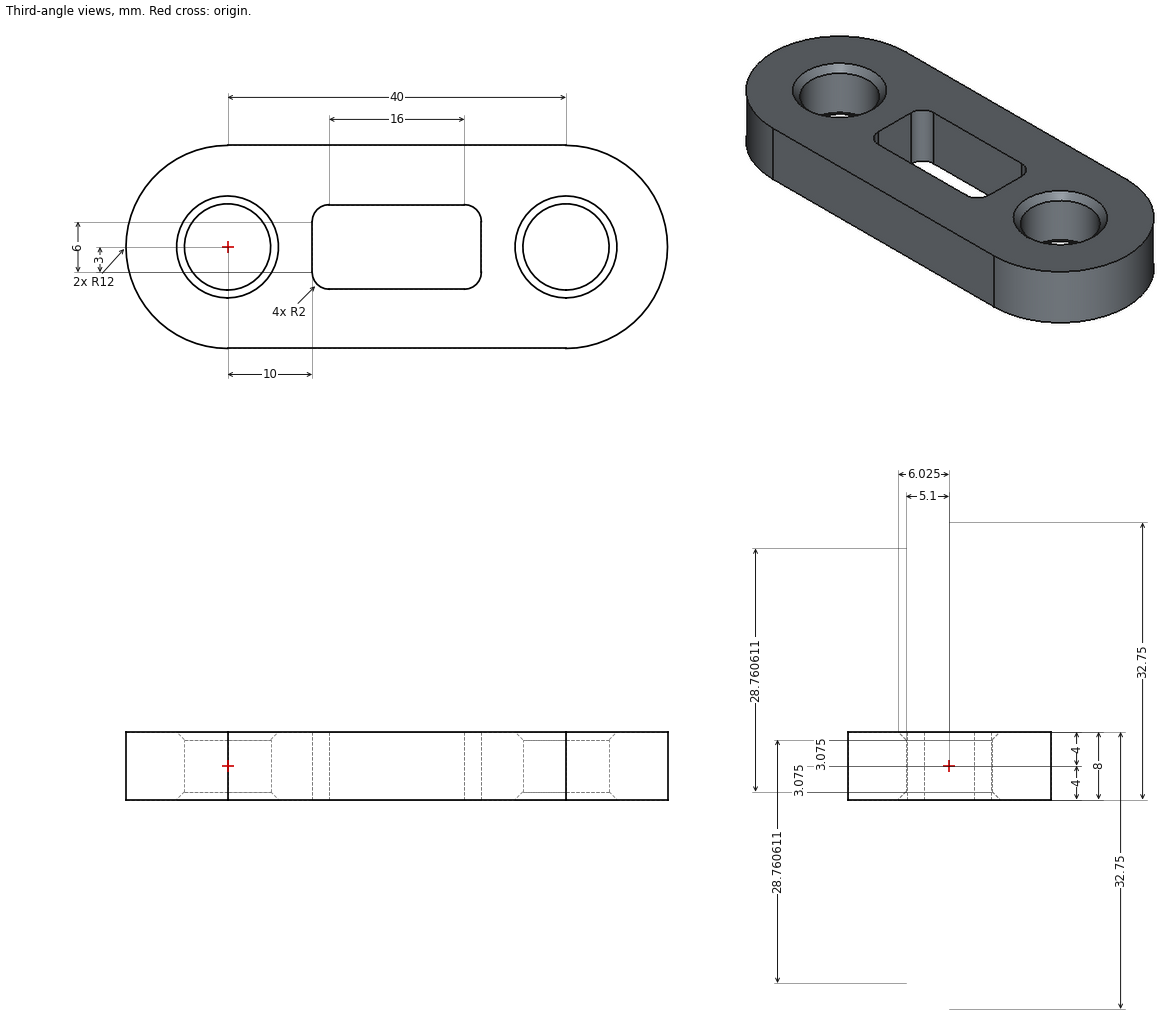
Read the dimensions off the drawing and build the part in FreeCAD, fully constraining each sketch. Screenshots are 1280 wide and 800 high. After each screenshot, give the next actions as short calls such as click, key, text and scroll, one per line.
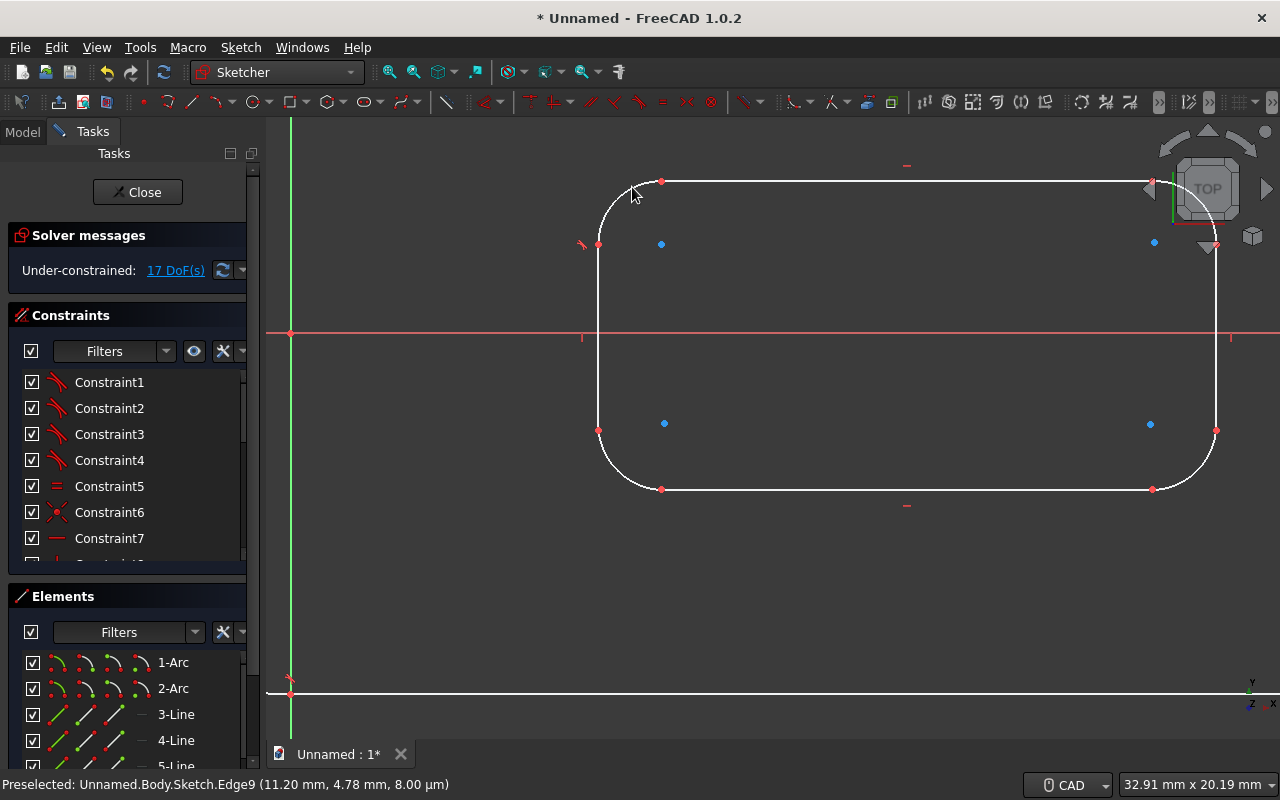
click(598, 374)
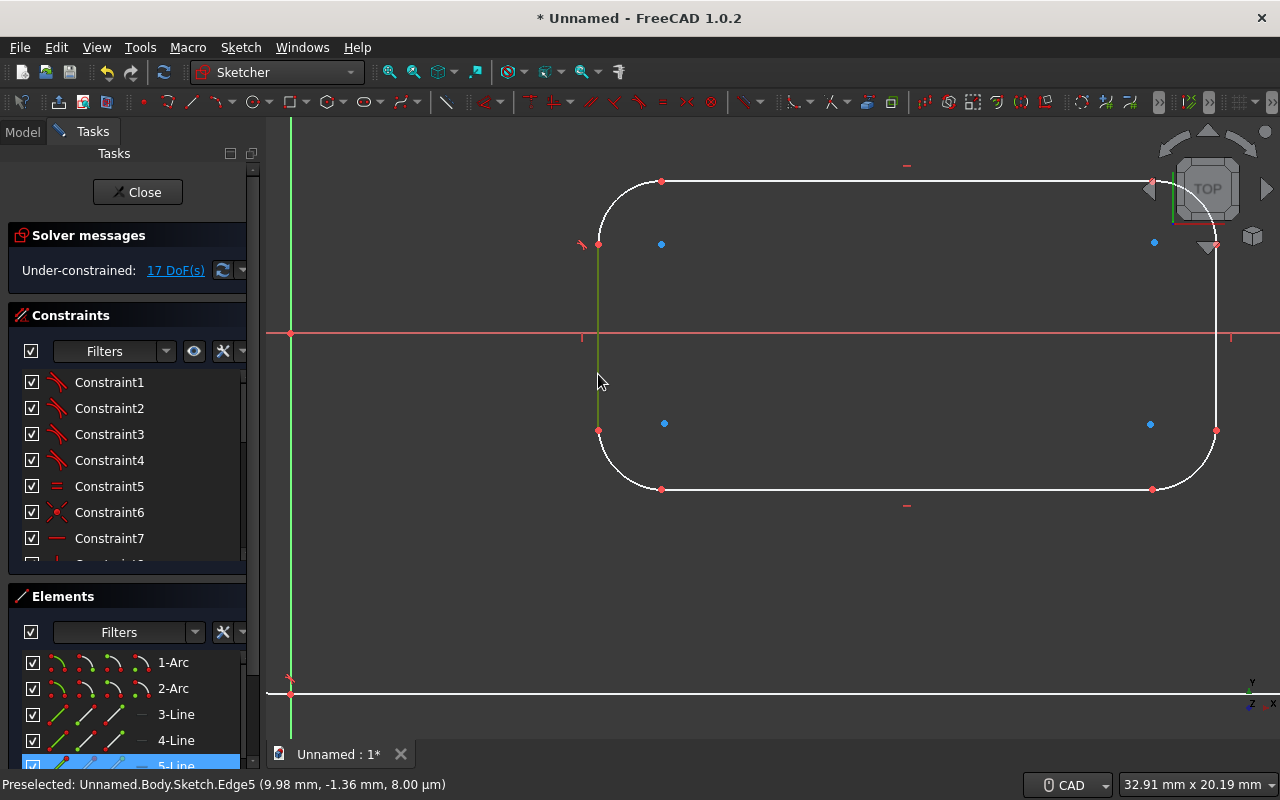
click(607, 457)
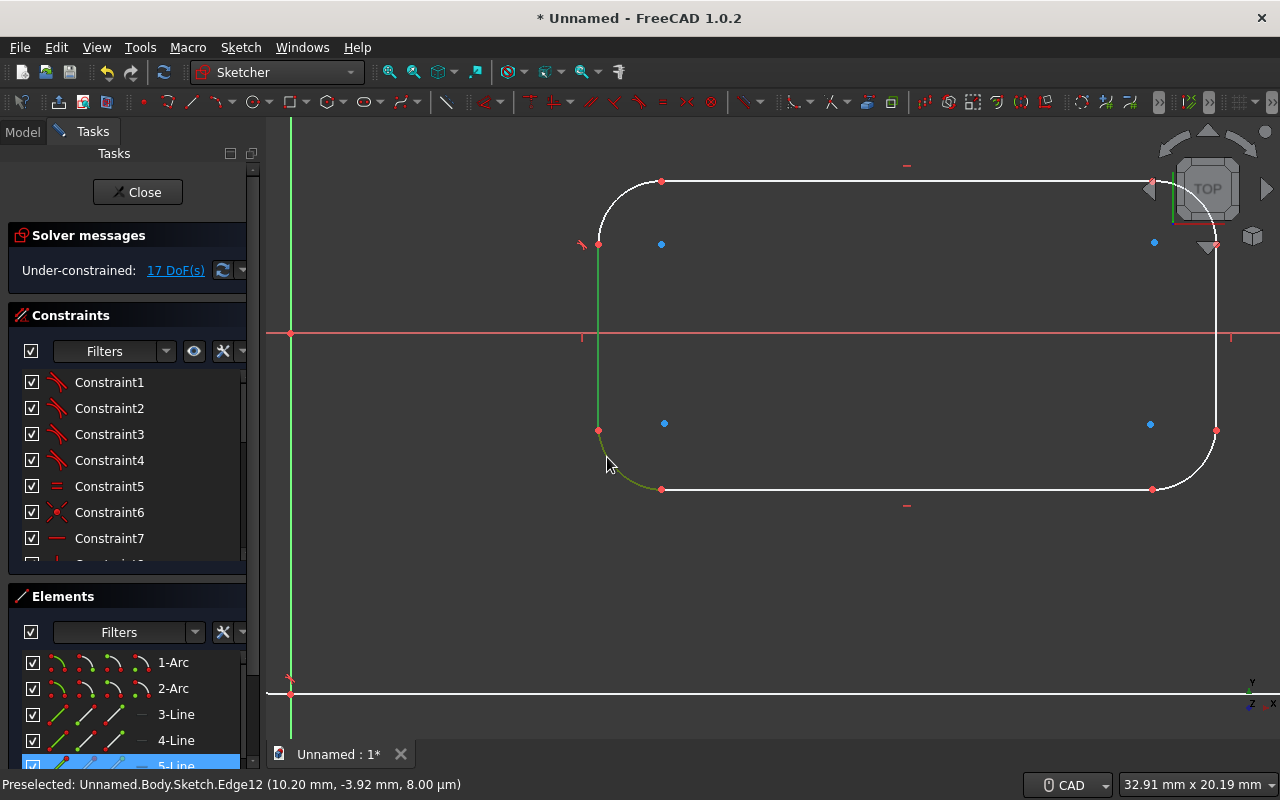
click(640, 102)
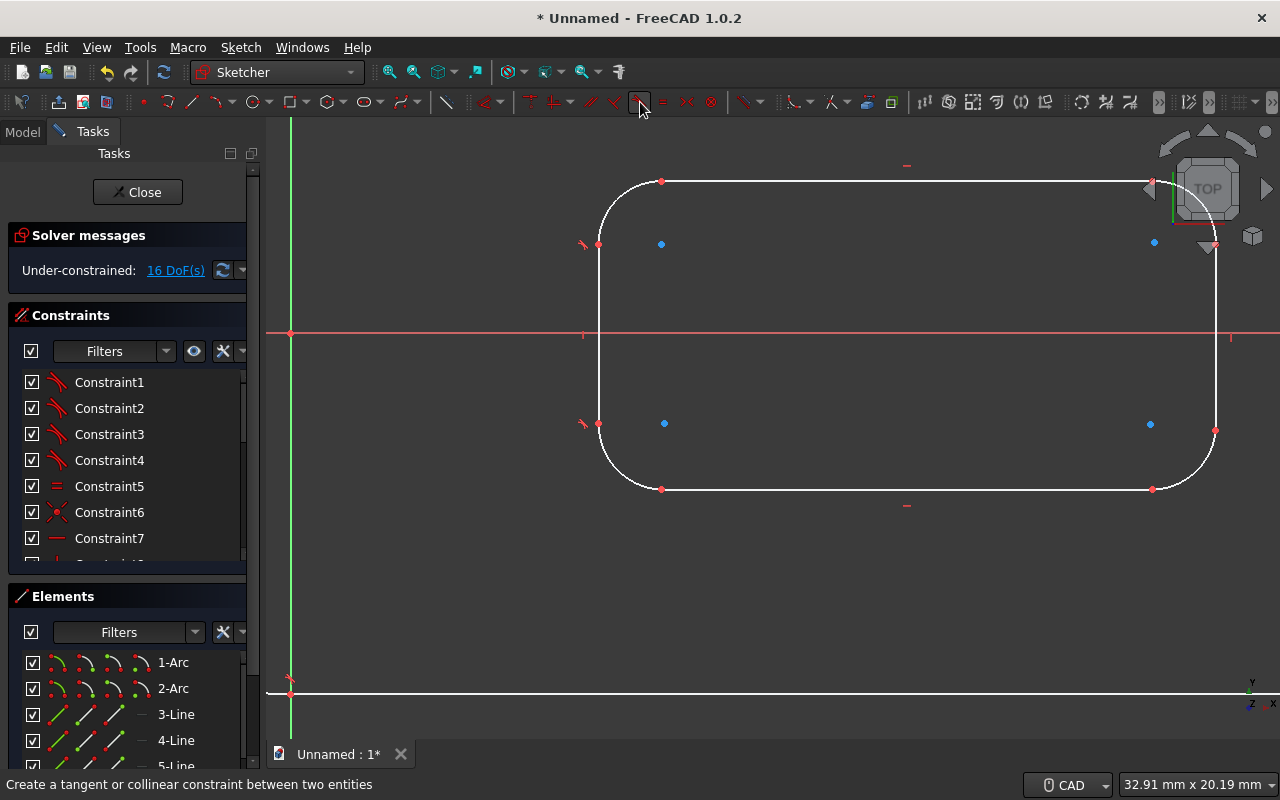
click(809, 181)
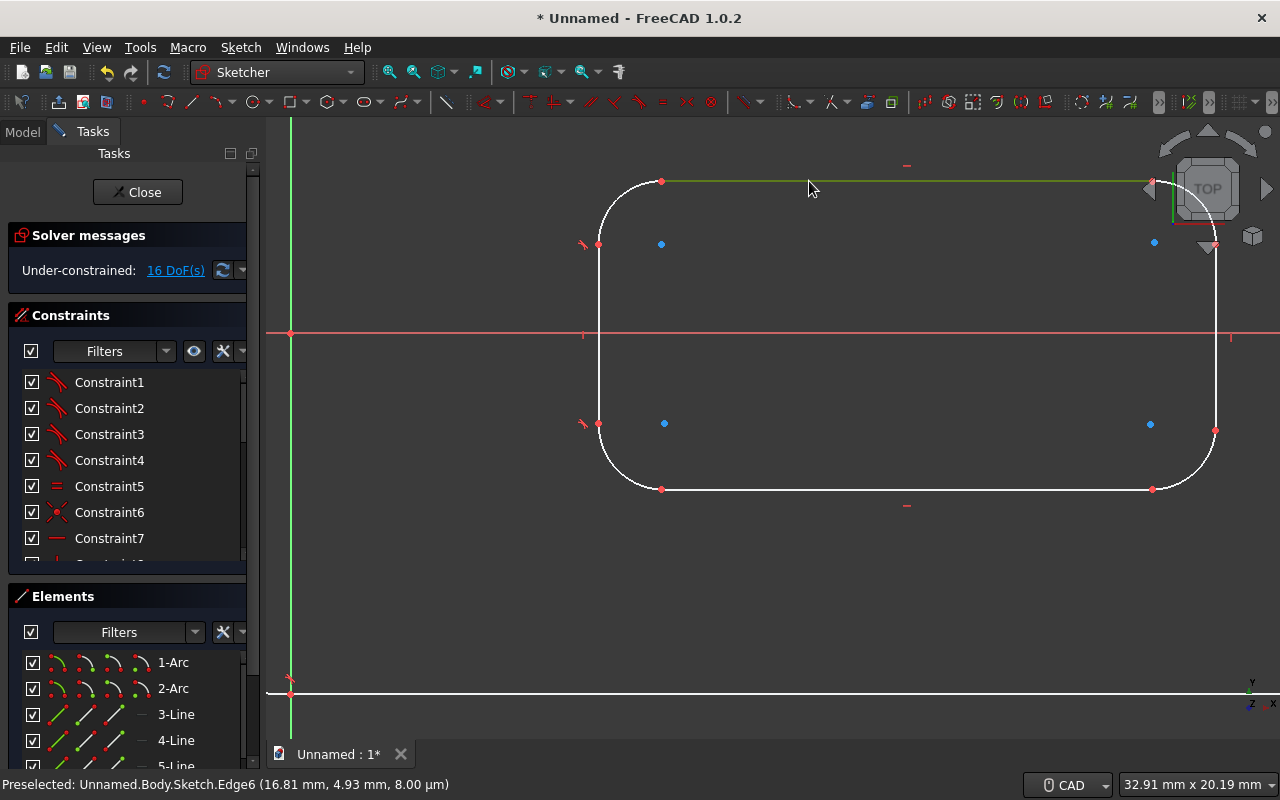
click(633, 188)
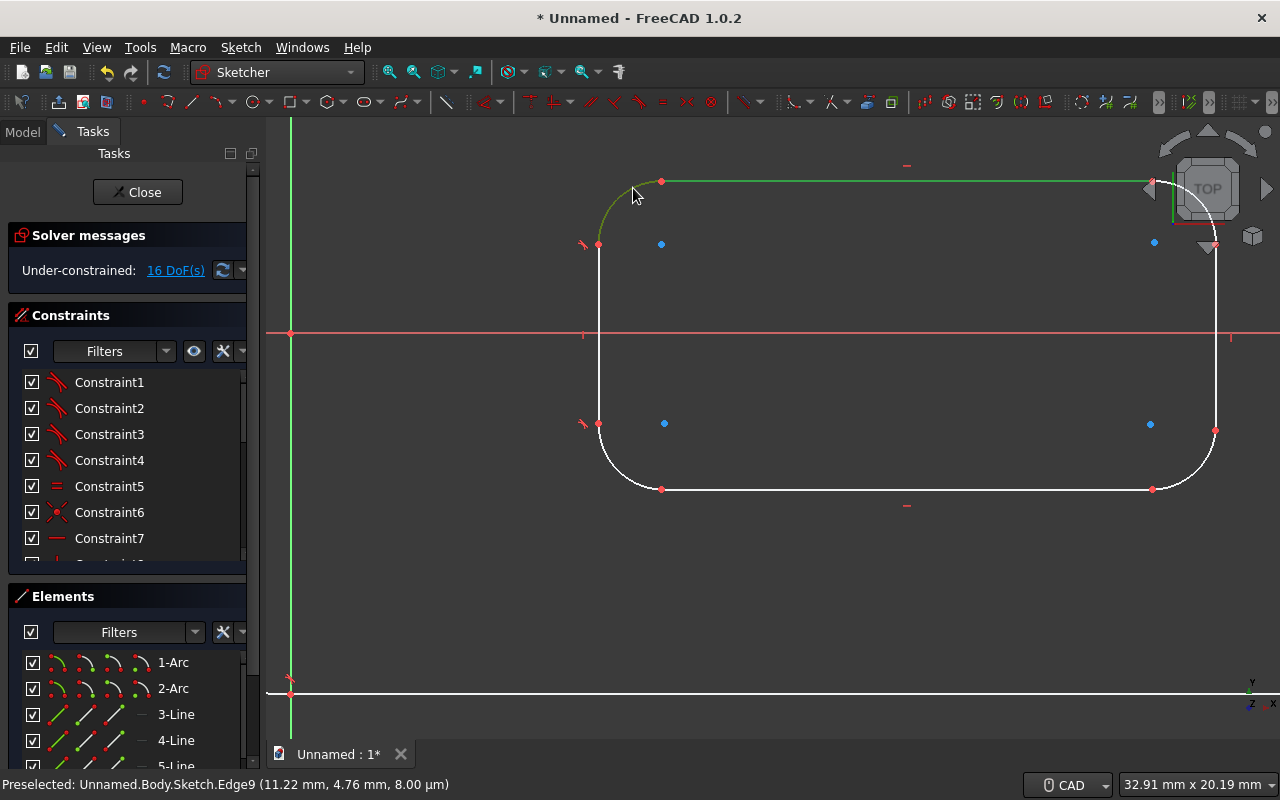
key(t)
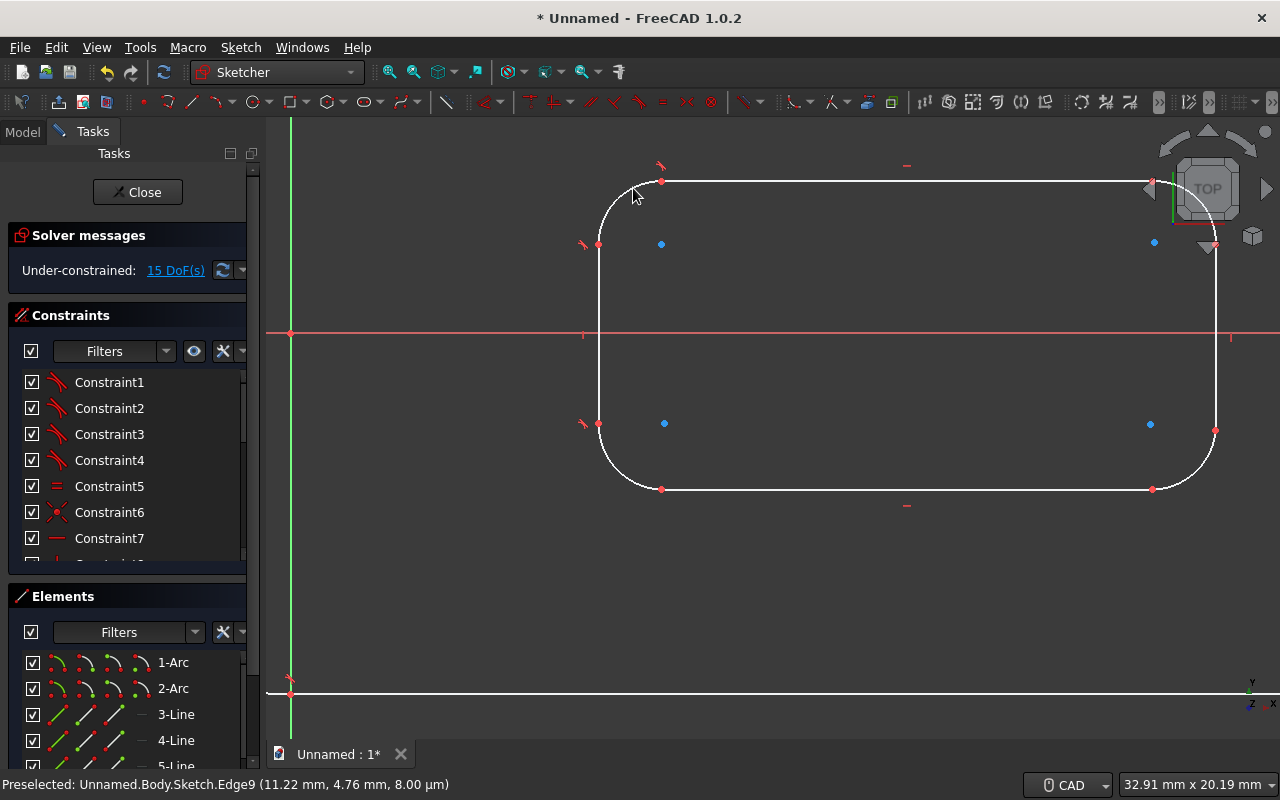
click(809, 181)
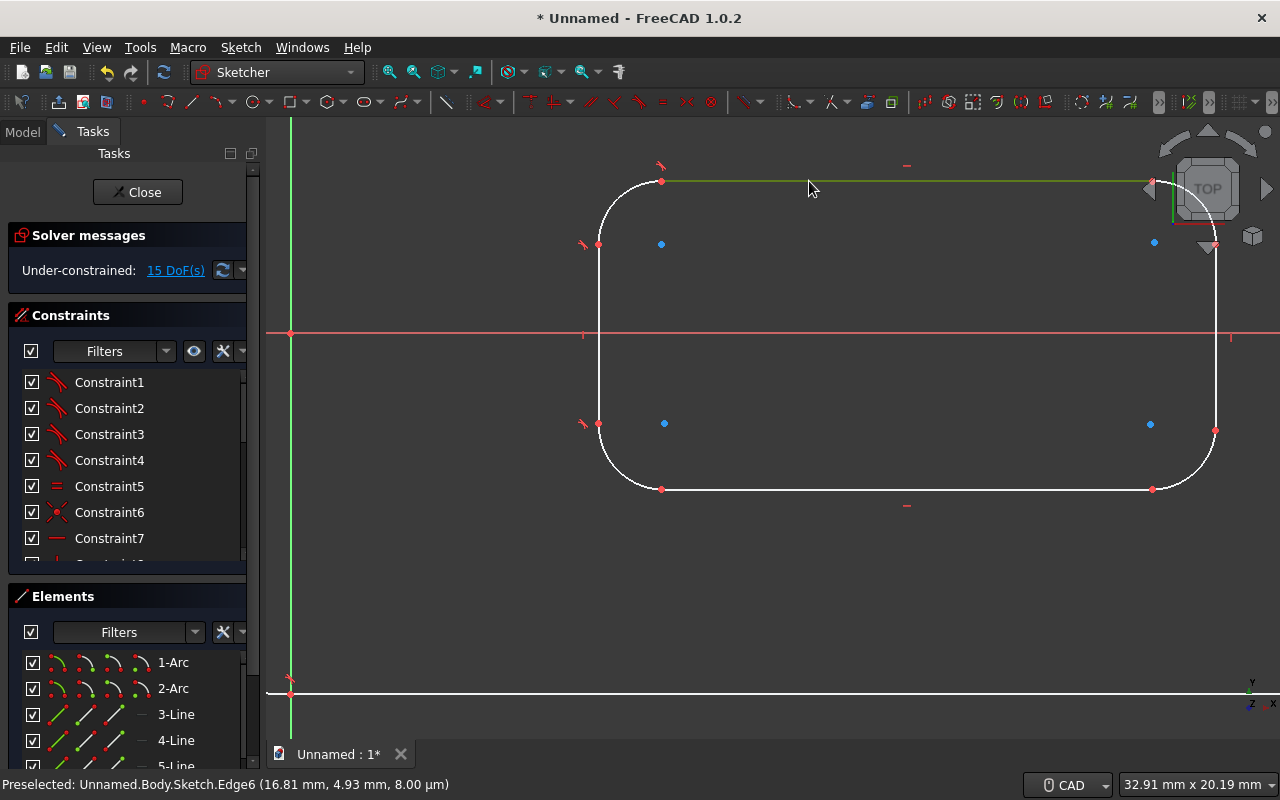
scroll(617, 469, down, 6)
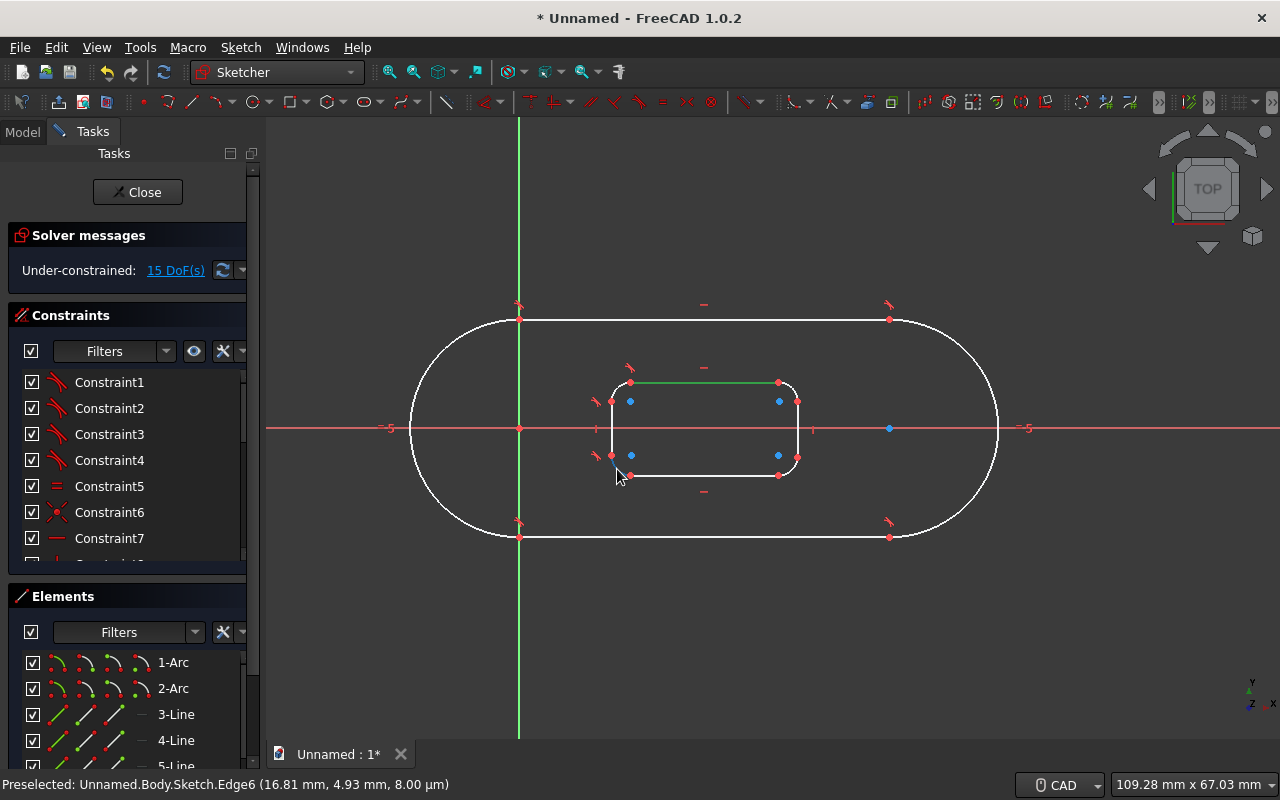
scroll(796, 393, up, 3)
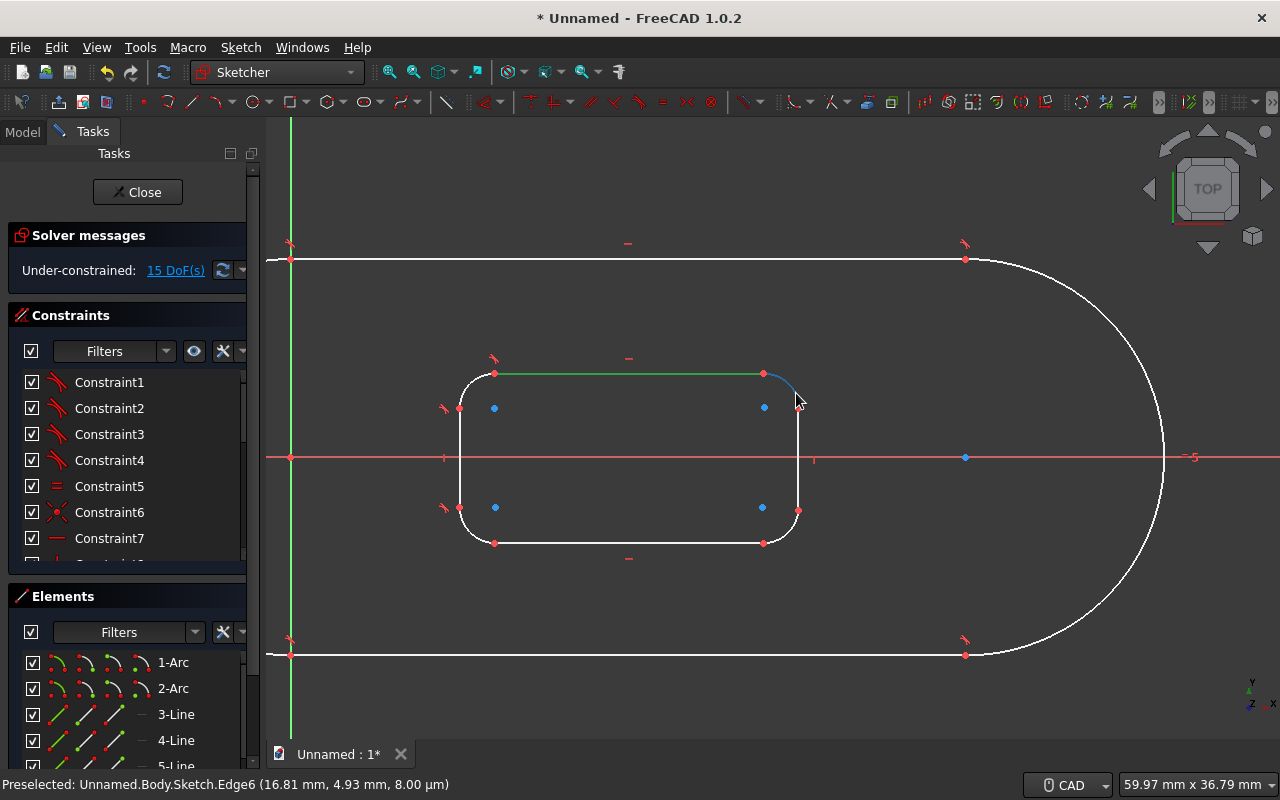
click(795, 393)